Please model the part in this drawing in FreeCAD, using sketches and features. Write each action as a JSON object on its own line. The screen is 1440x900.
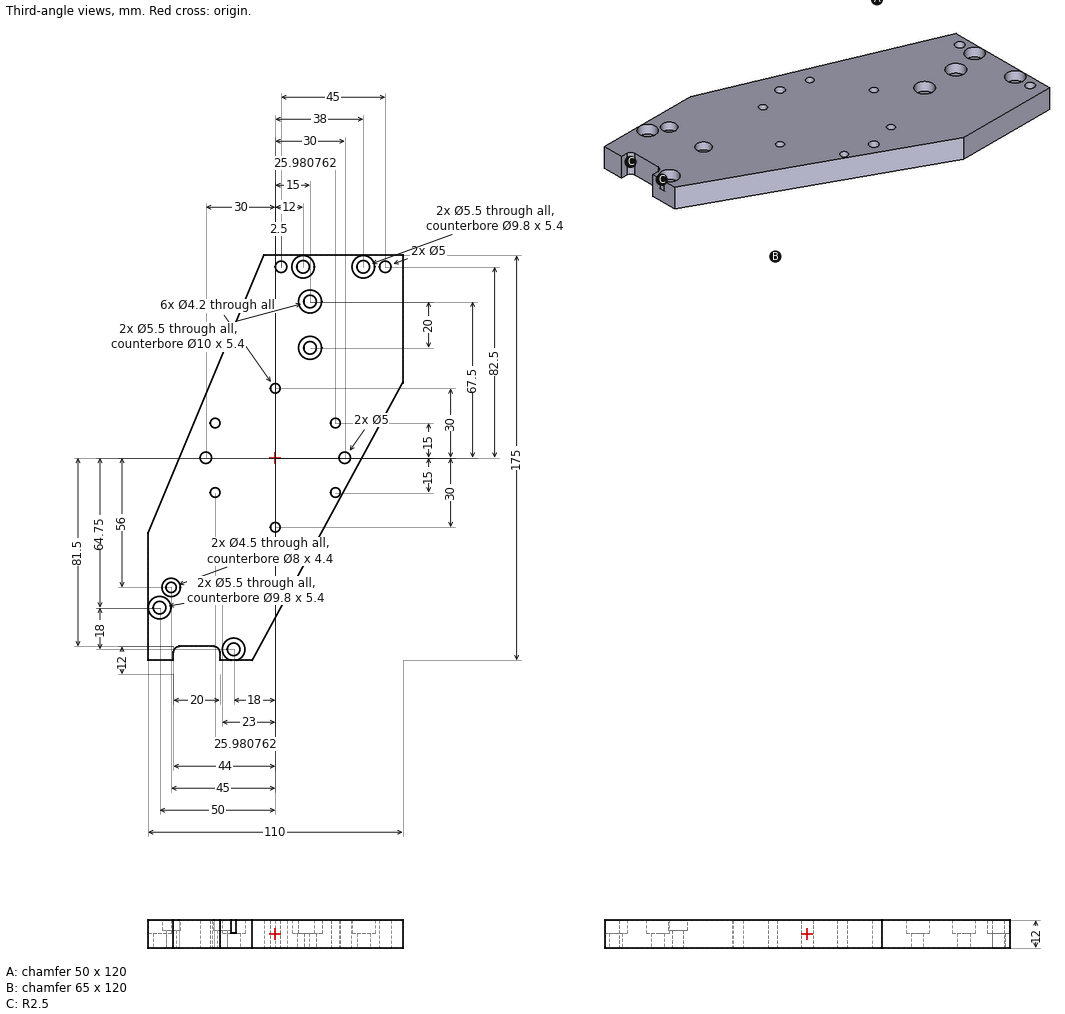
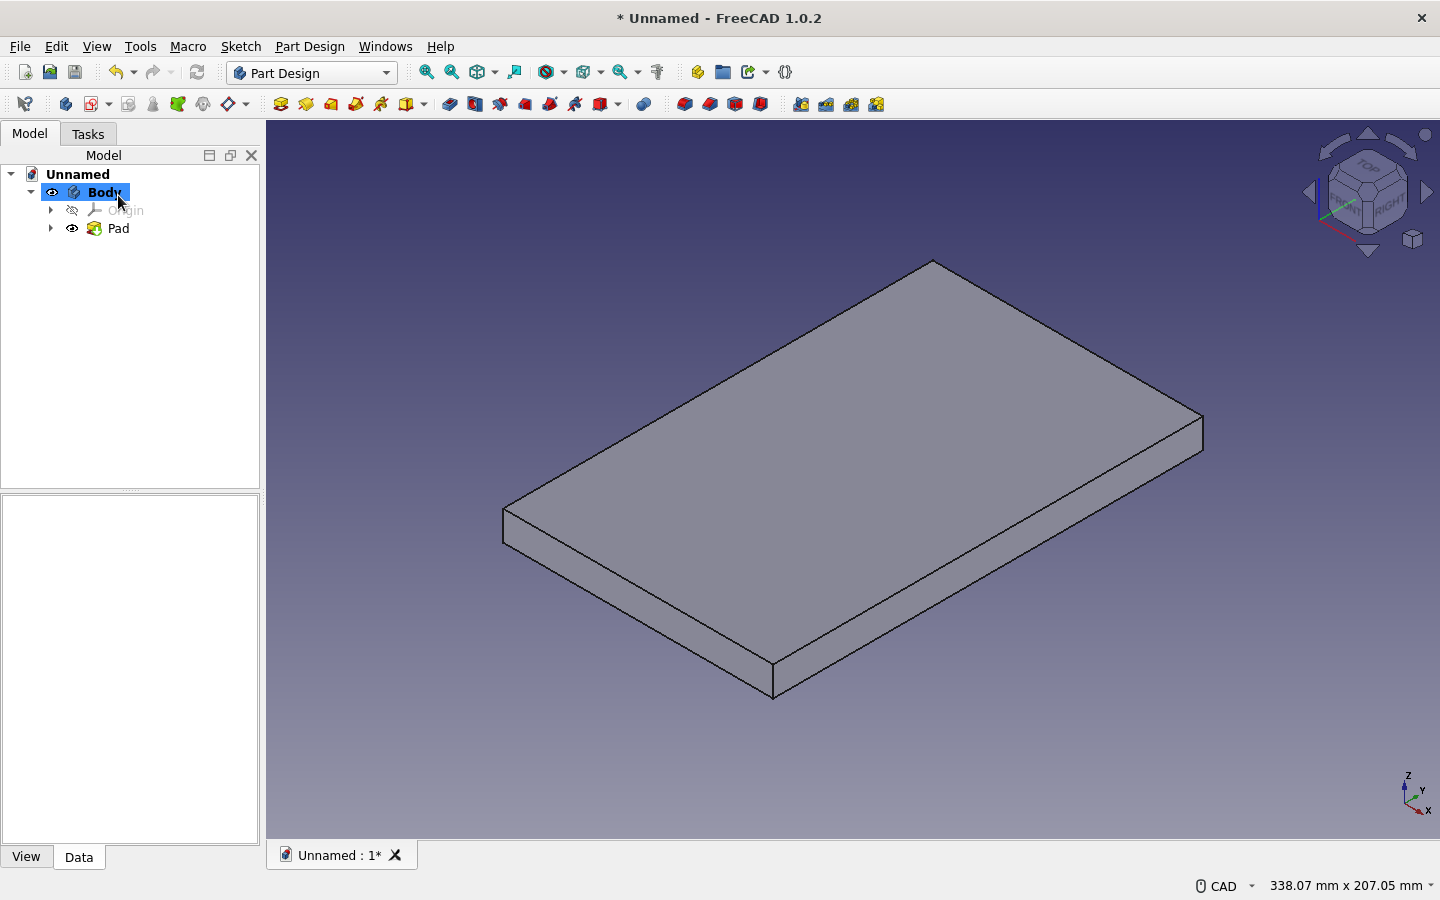
{"action": "key", "text": "2"}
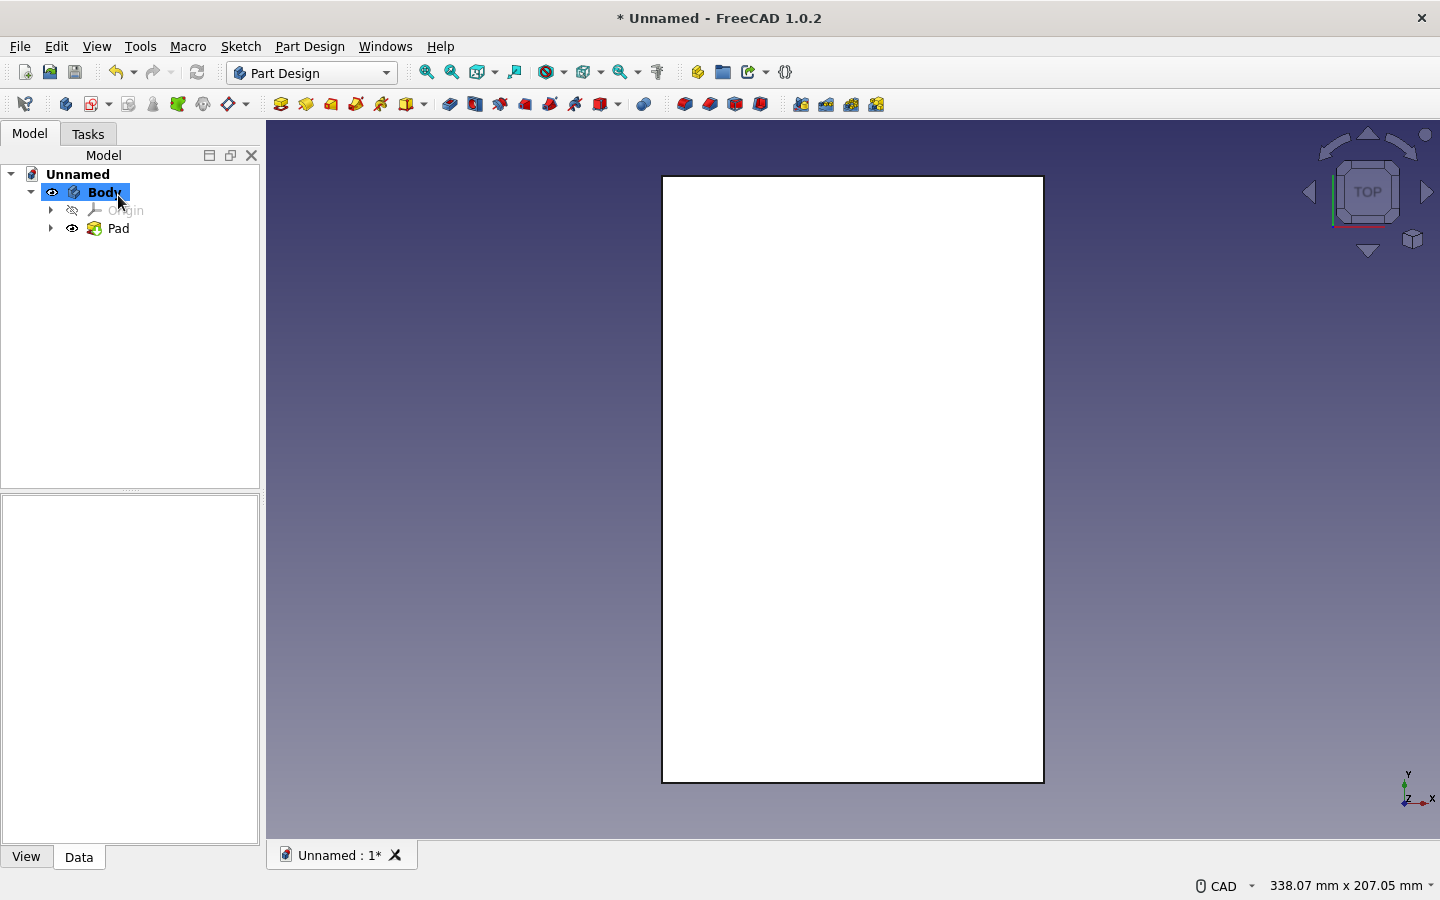
{"action": "key", "text": "1"}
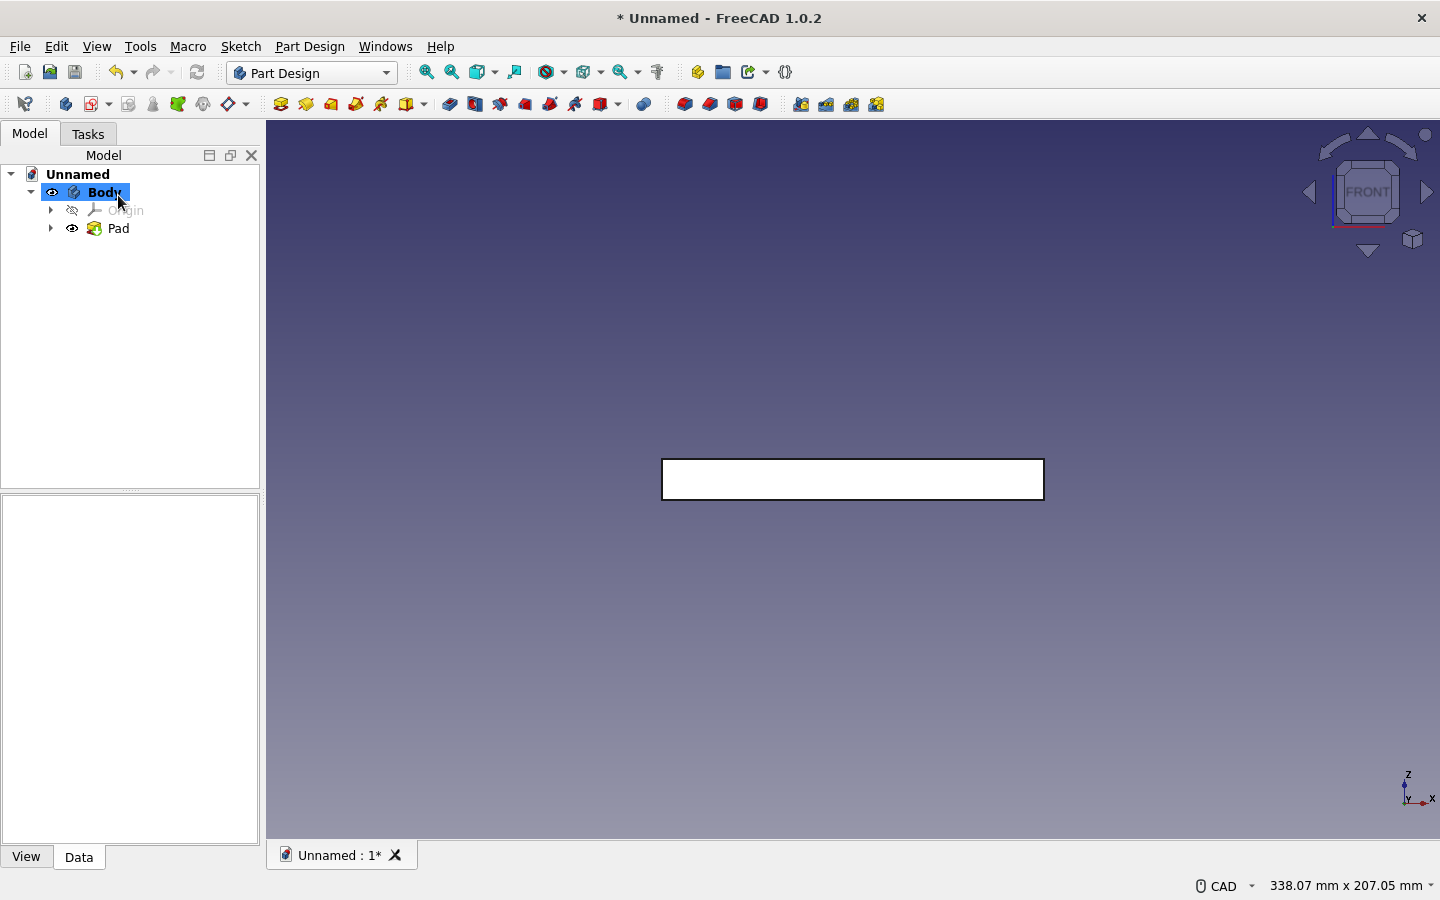
{"action": "key", "text": "v f"}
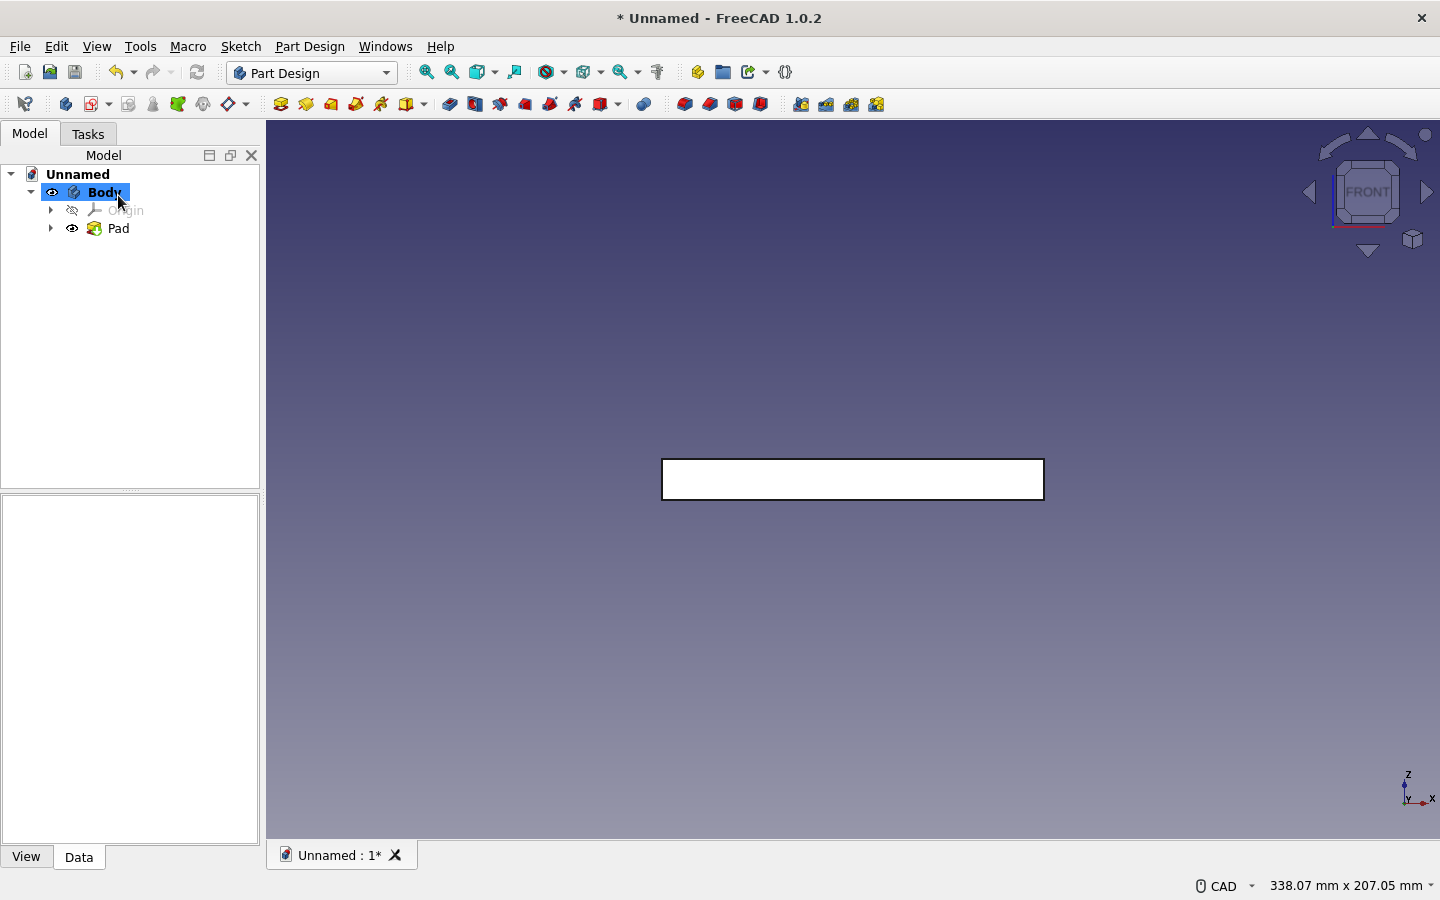
{"action": "key", "text": "3"}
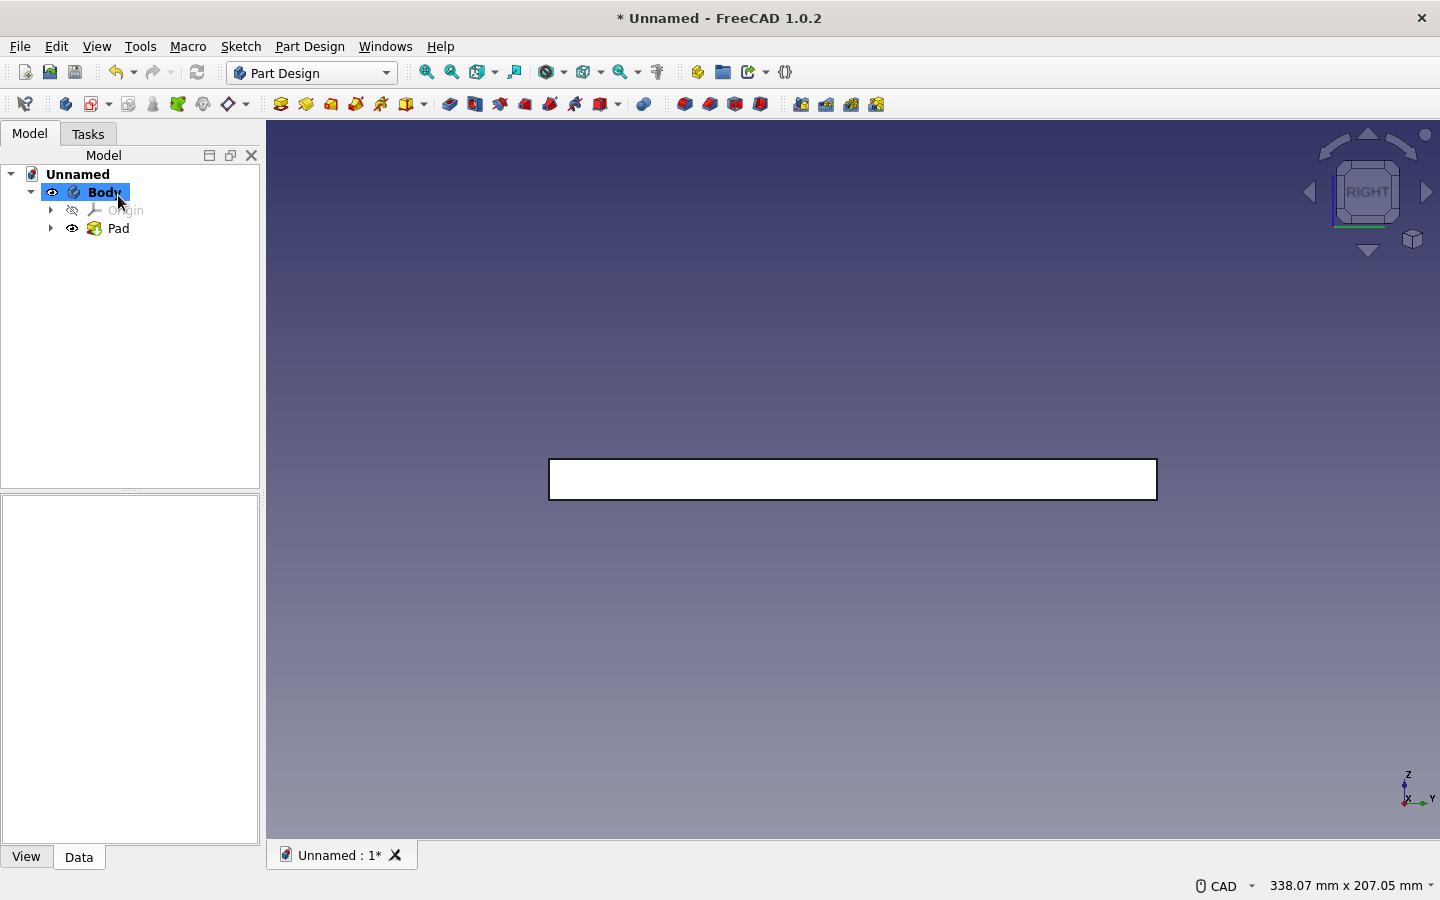
{"action": "key", "text": "5"}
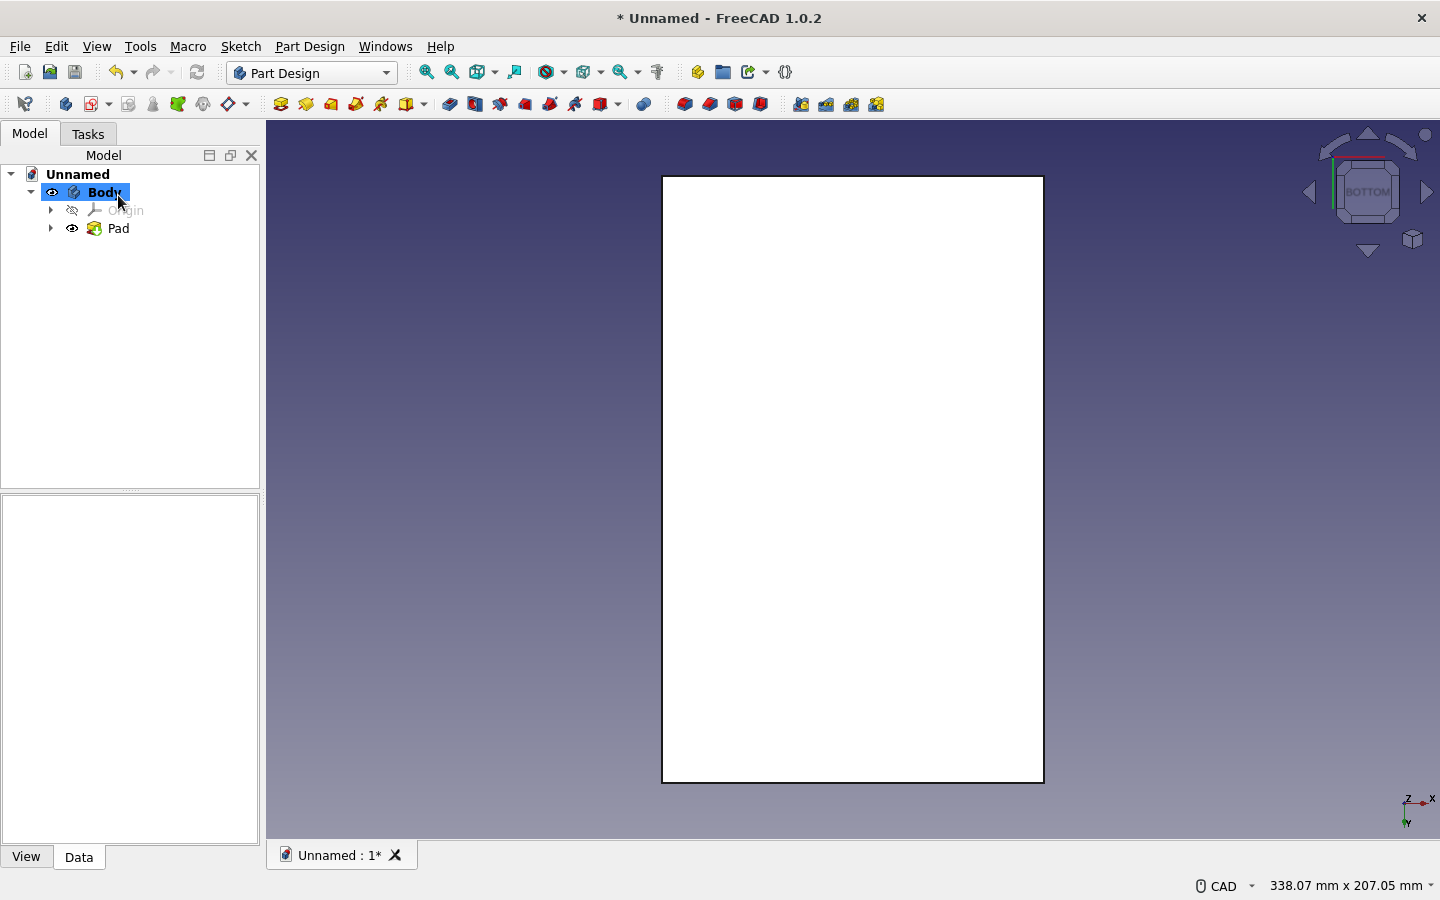
{"action": "key", "text": "4"}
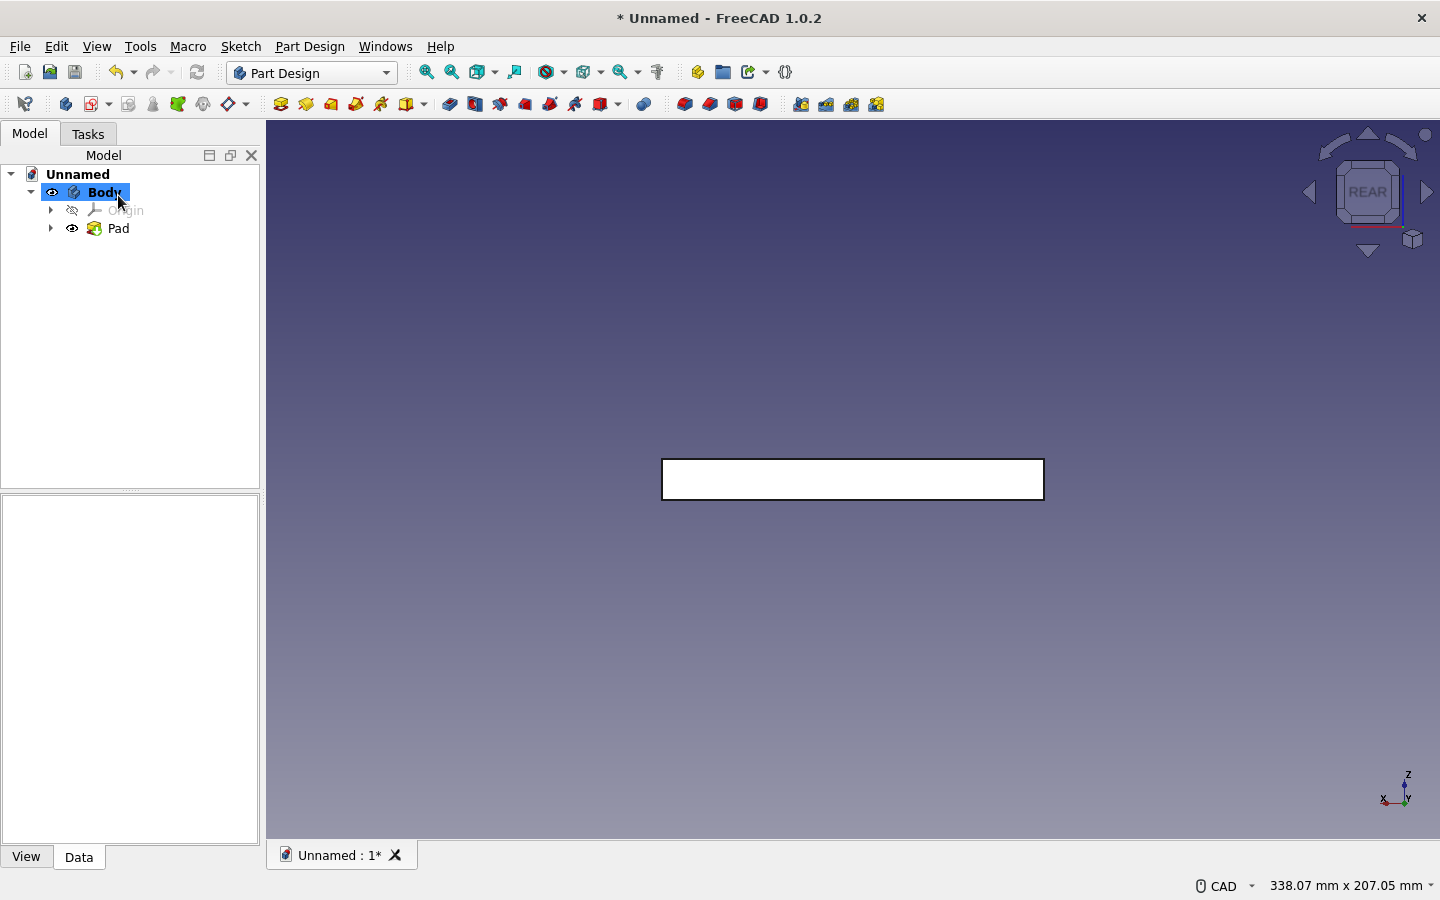
{"action": "key", "text": "v f"}